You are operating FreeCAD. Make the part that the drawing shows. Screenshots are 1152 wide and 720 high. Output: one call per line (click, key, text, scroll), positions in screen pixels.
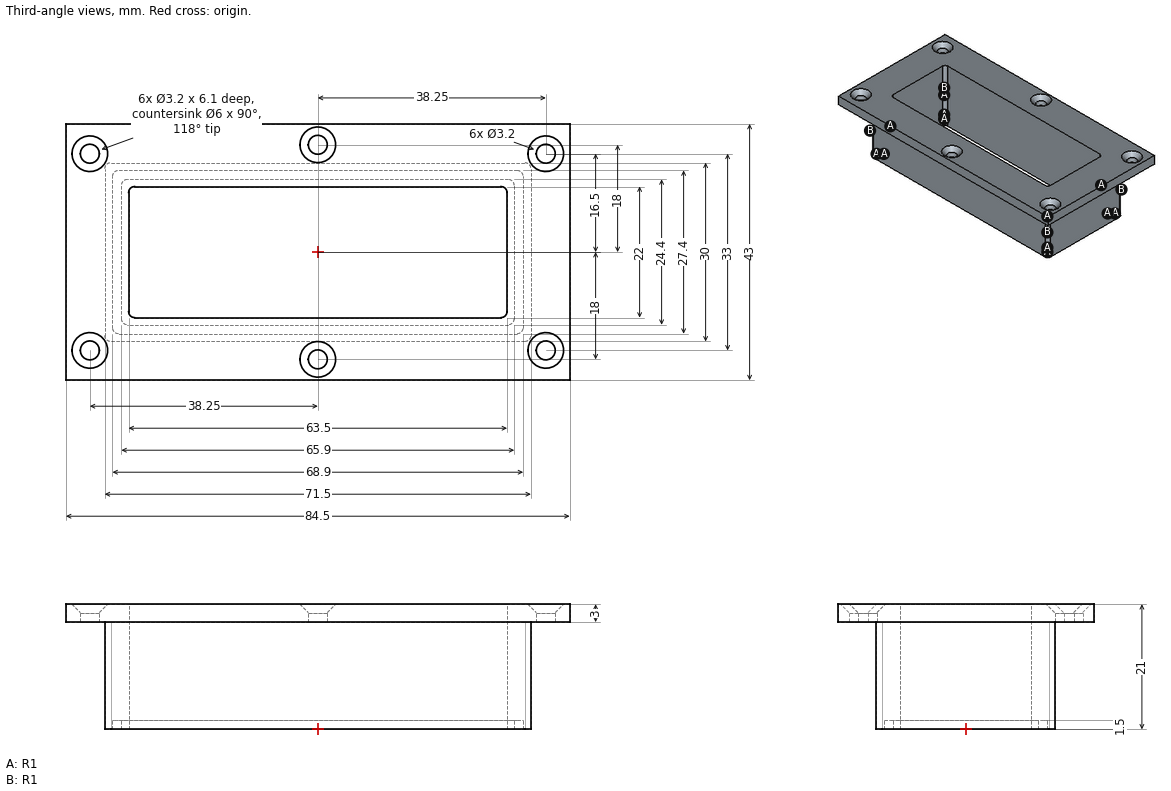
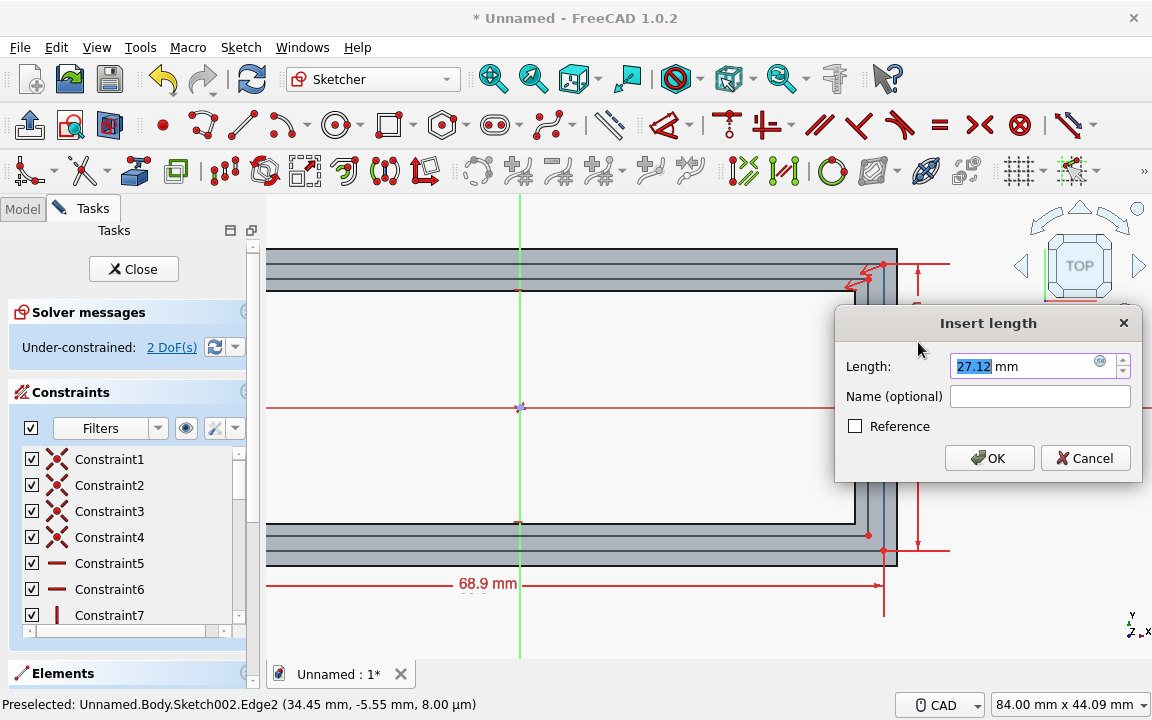
text(27.4)
key(Return)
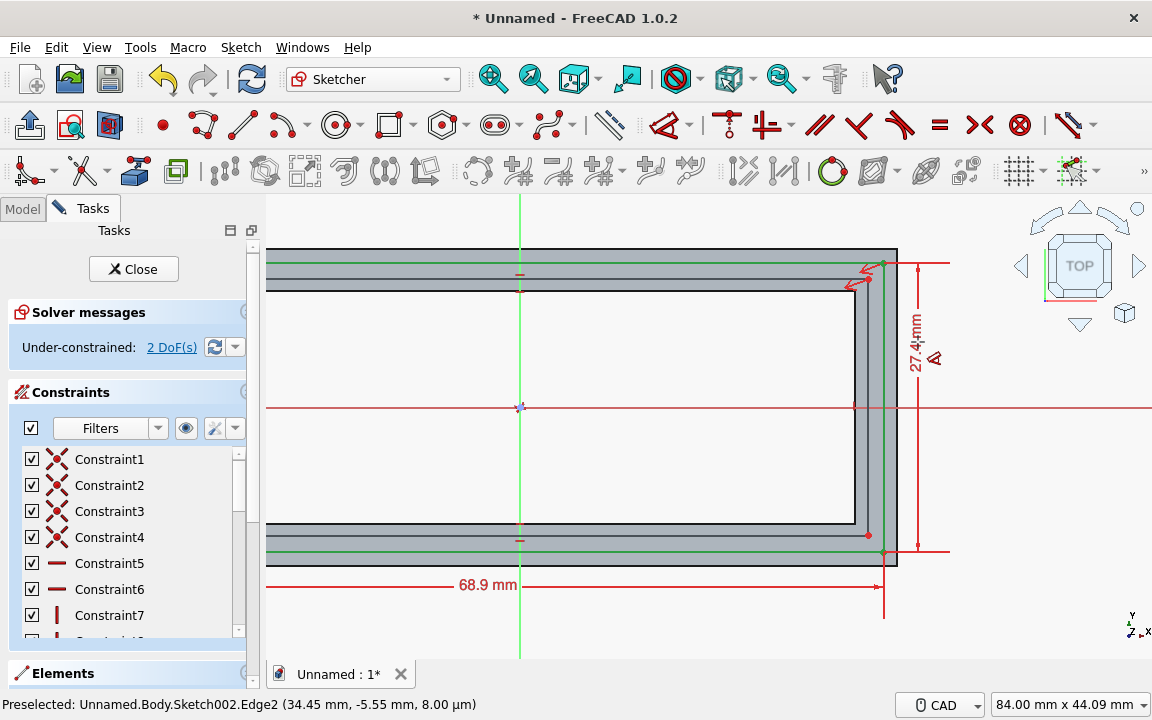
click(381, 536)
click(581, 570)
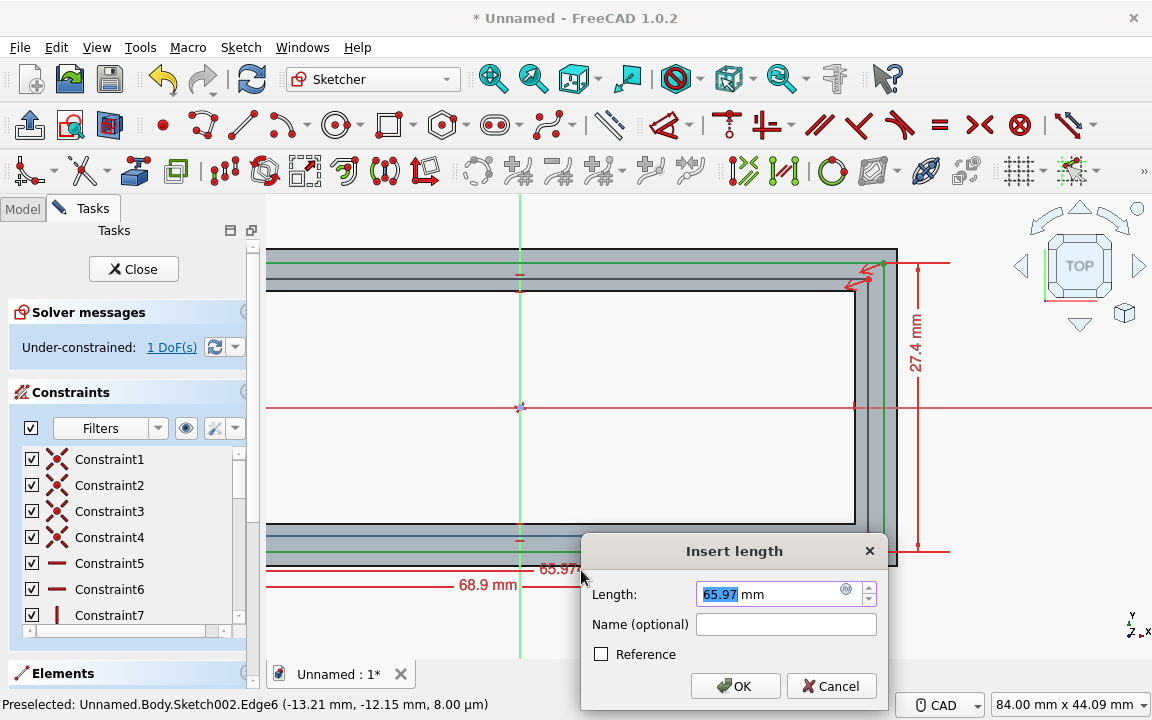
text(65.9)
key(Return)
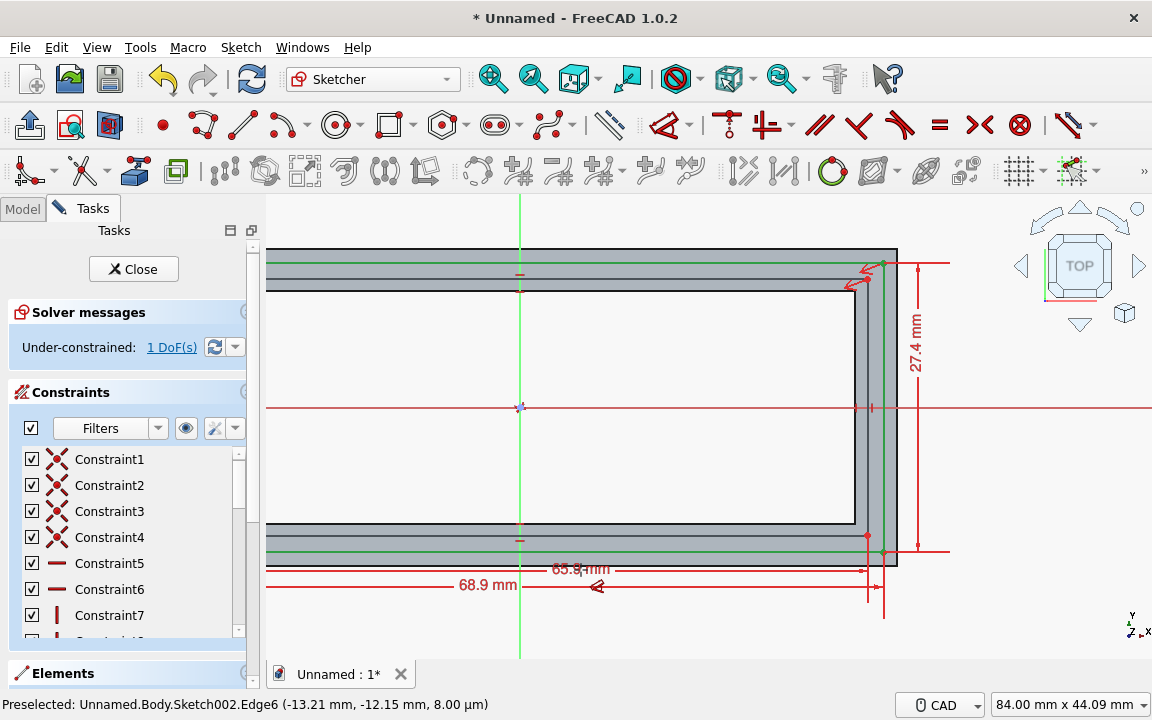
click(868, 459)
click(902, 466)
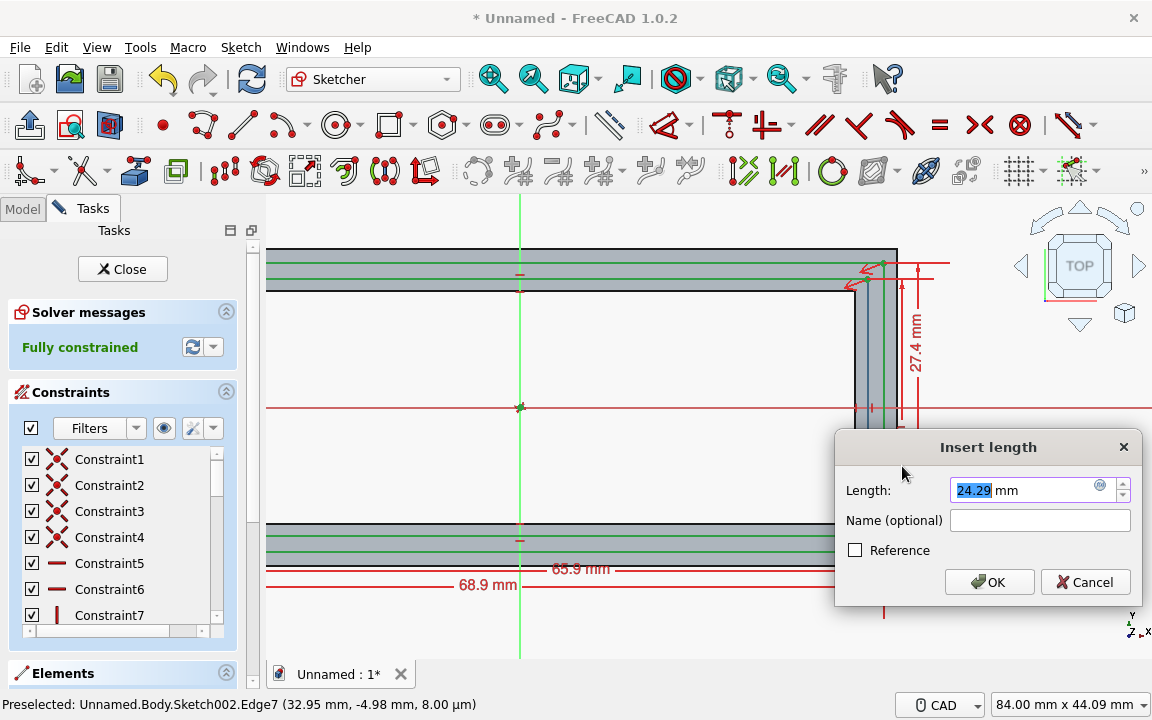
text(24.4)
key(Return)
key(Escape)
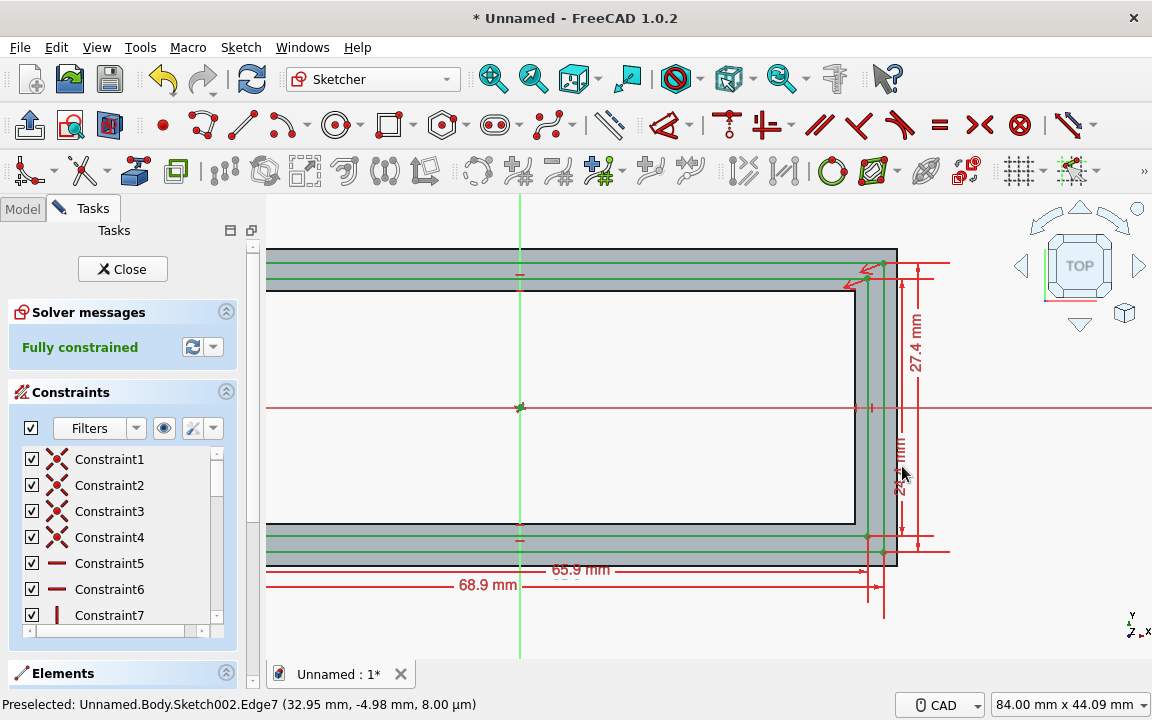
click(123, 269)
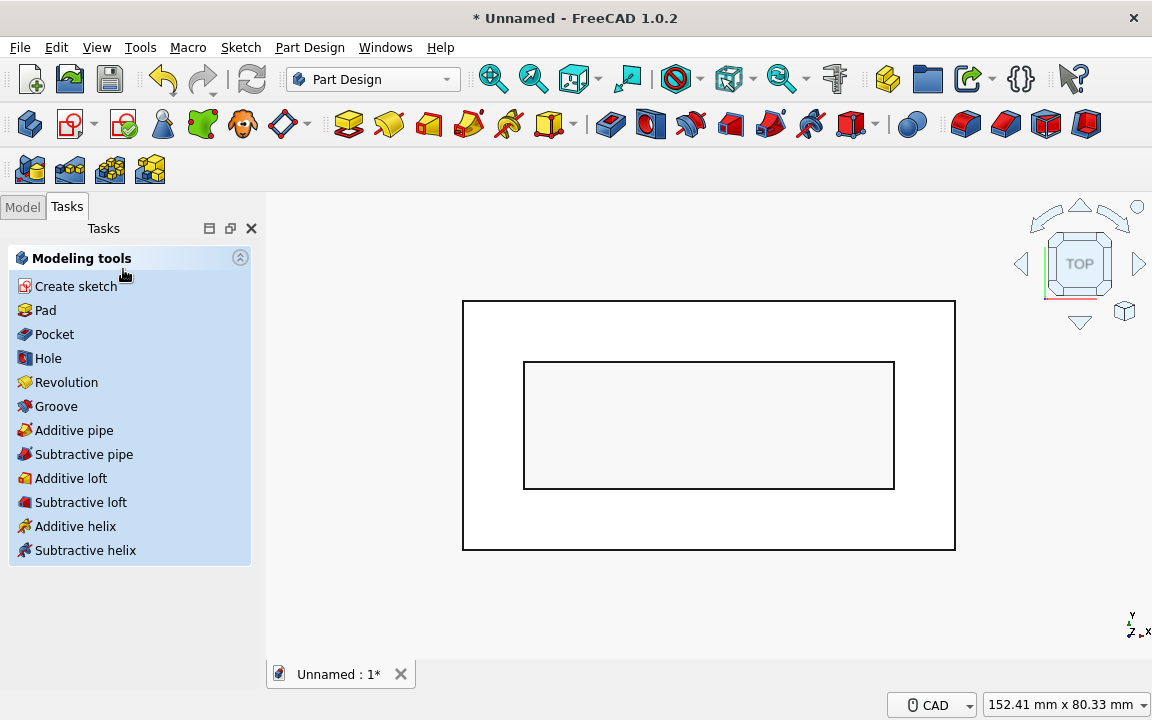
click(612, 124)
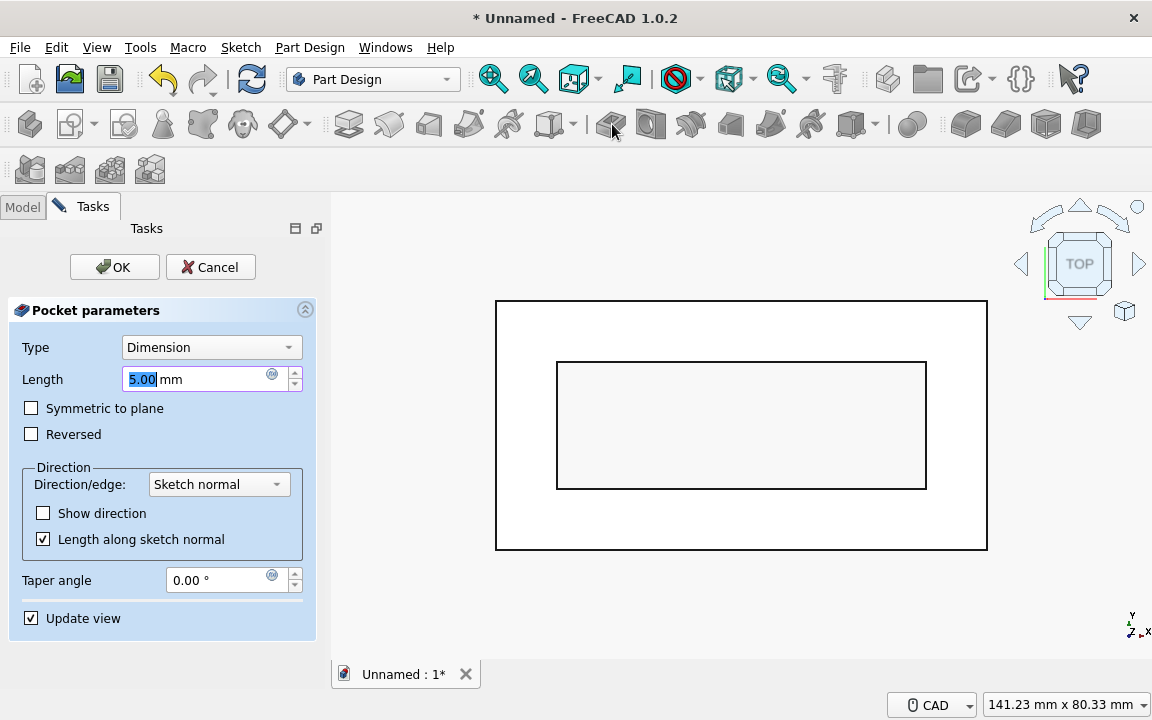
text(1.5)
key(Tab)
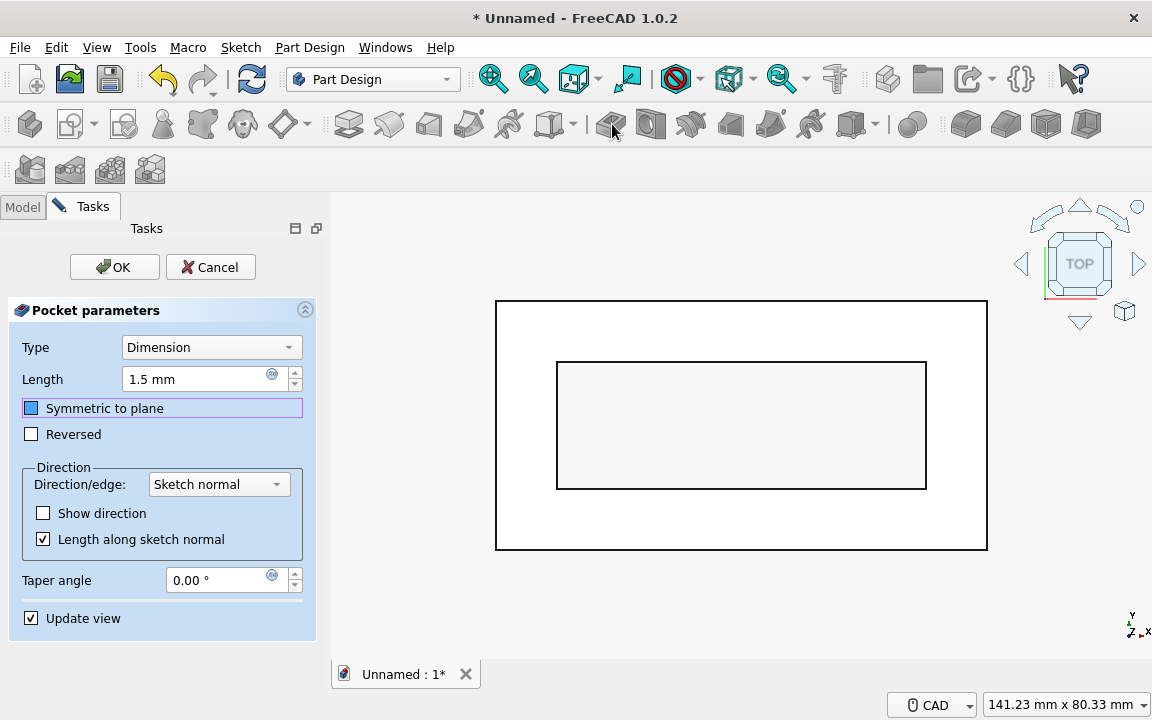
click(30, 434)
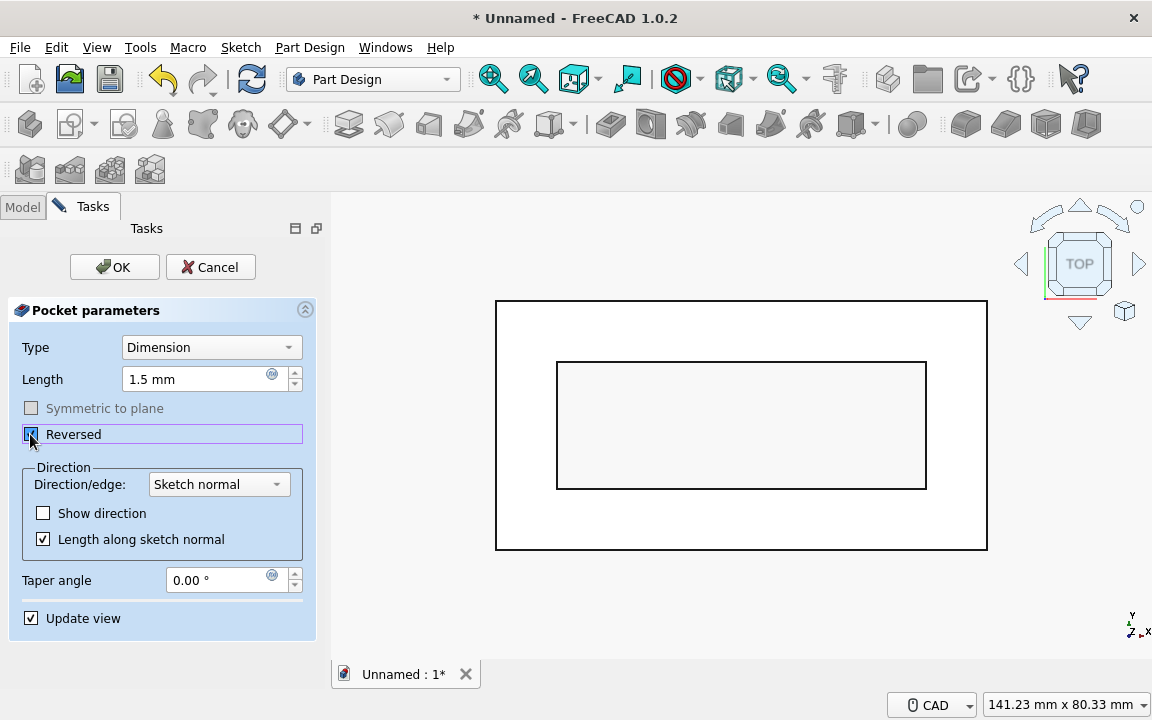
click(115, 267)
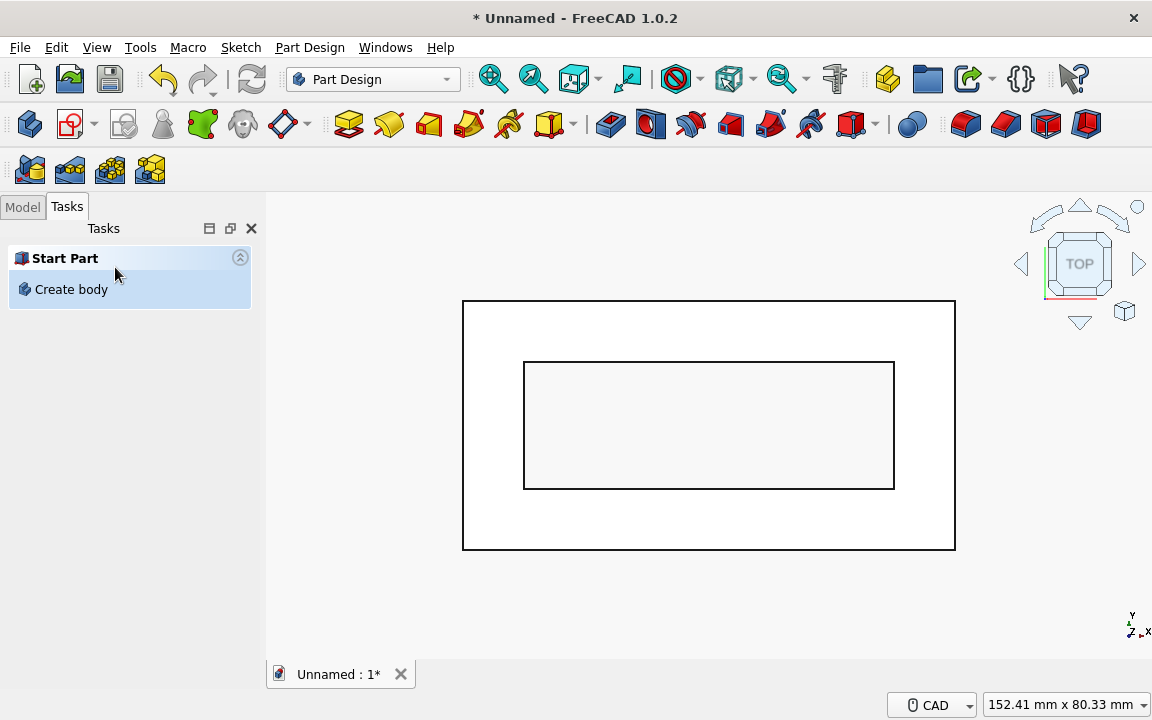
key(5)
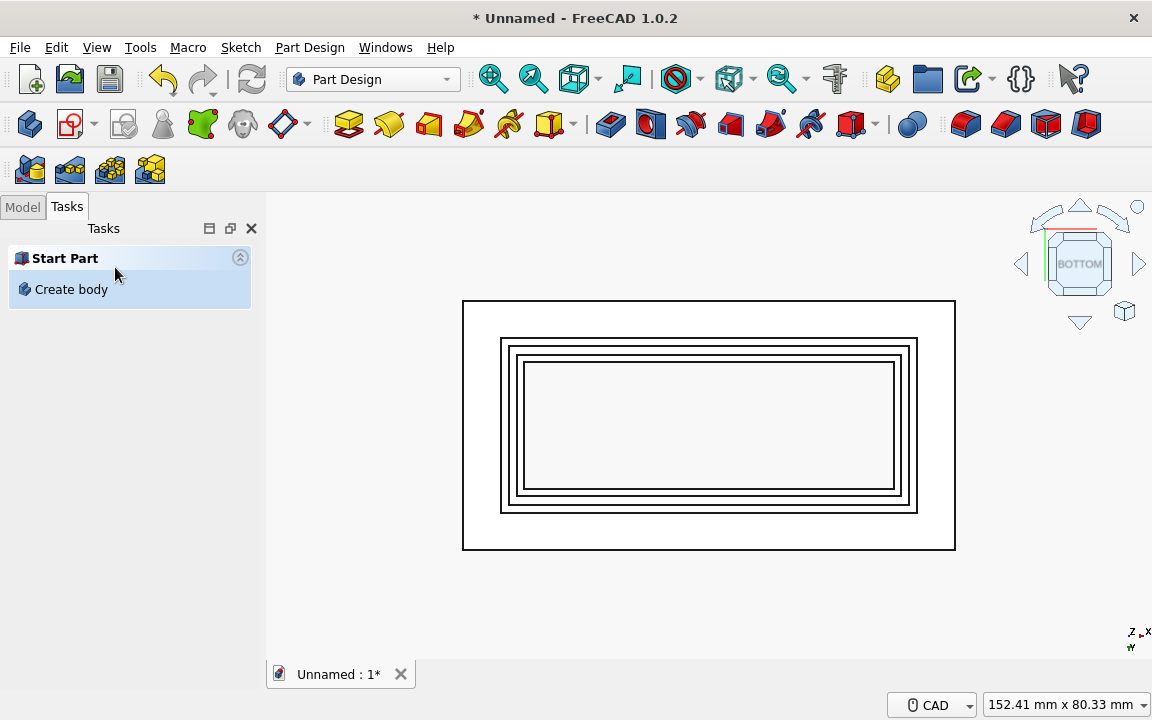
click(920, 317)